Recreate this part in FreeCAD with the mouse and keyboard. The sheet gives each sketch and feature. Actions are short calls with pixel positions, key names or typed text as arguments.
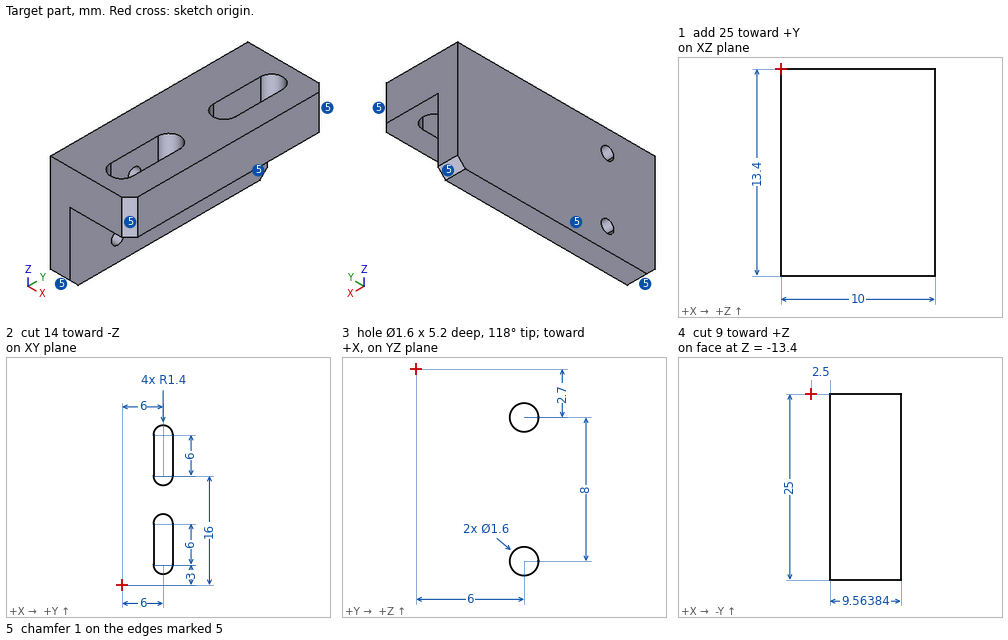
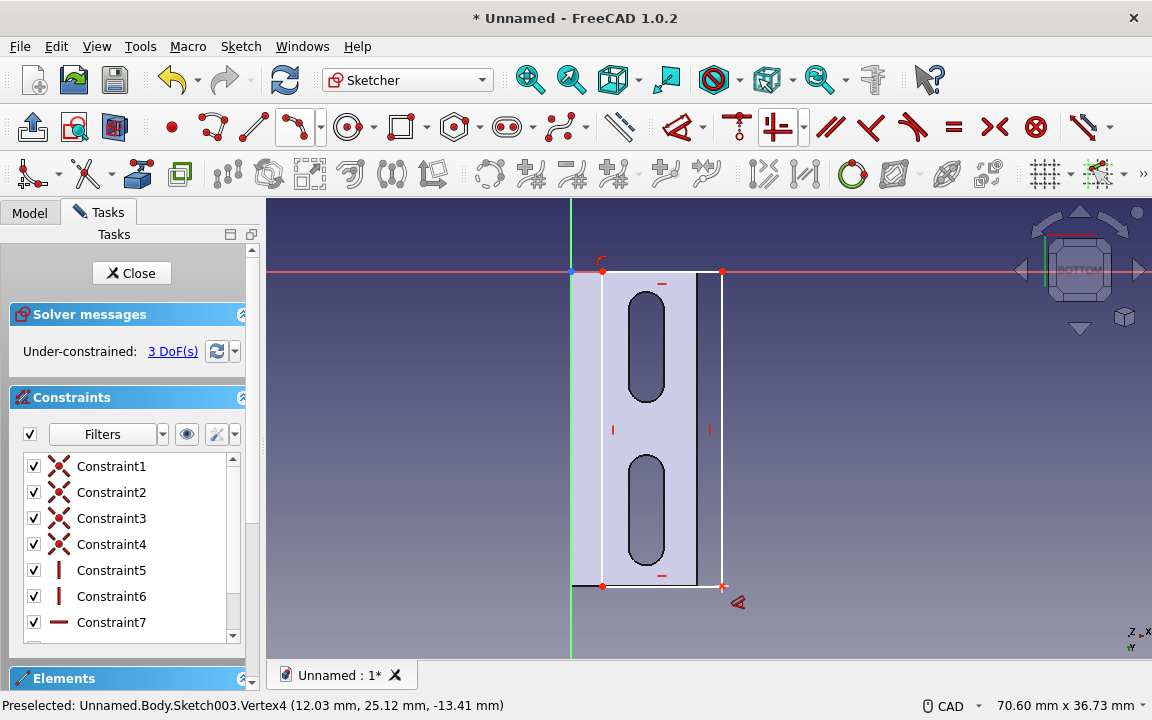
click(602, 366)
click(636, 429)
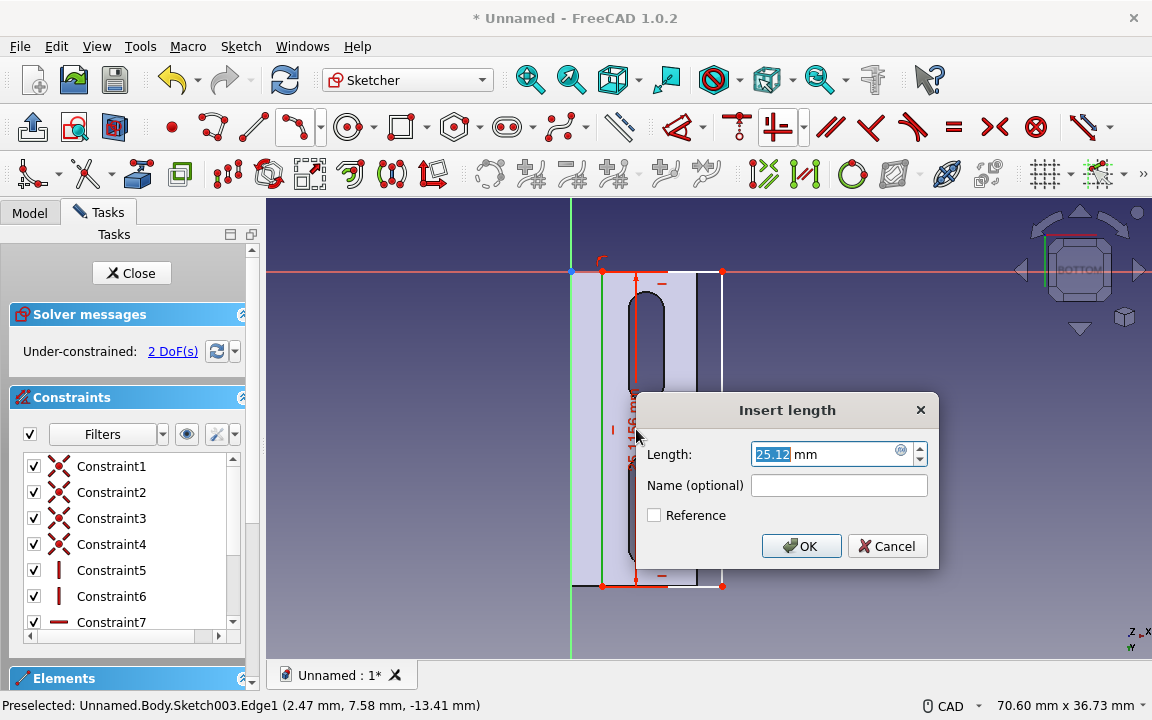
text(25)
key(Return)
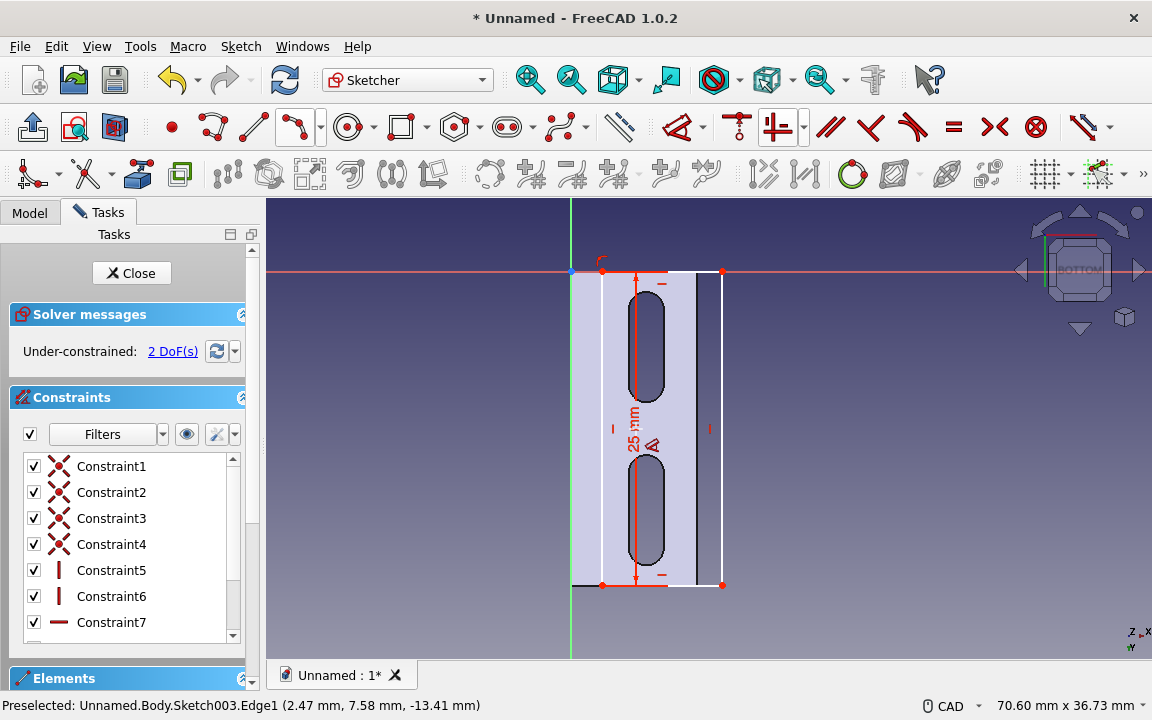
scroll(602, 272, up, 2)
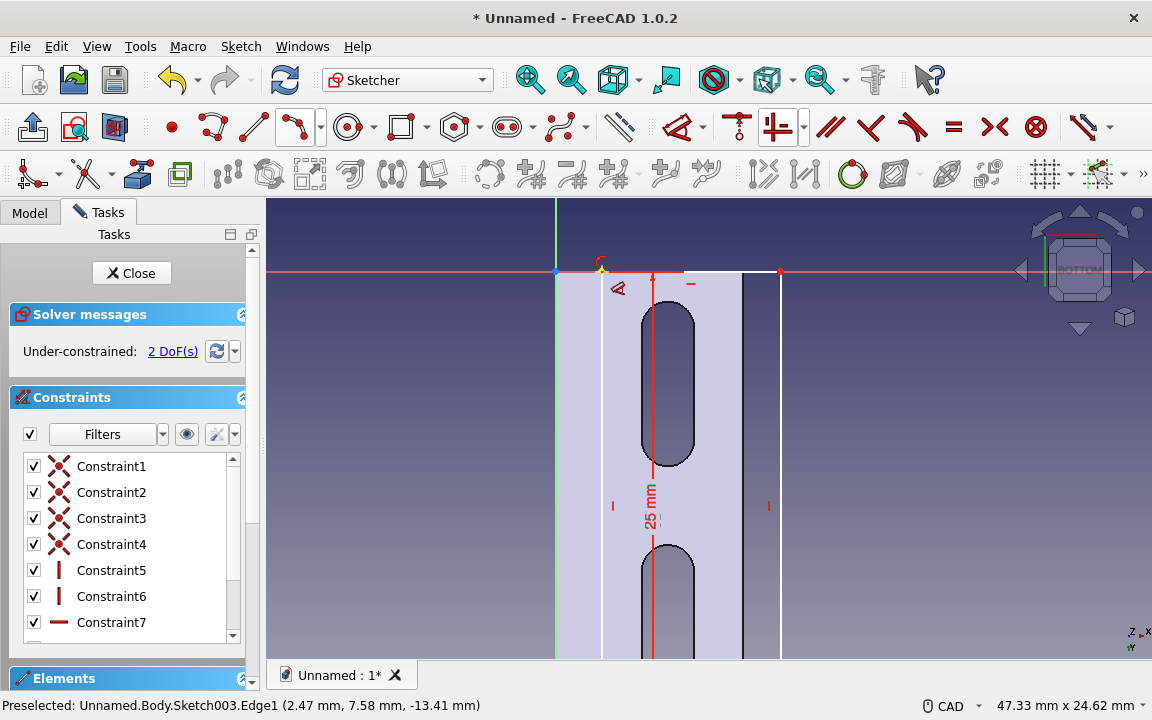
click(602, 272)
click(579, 238)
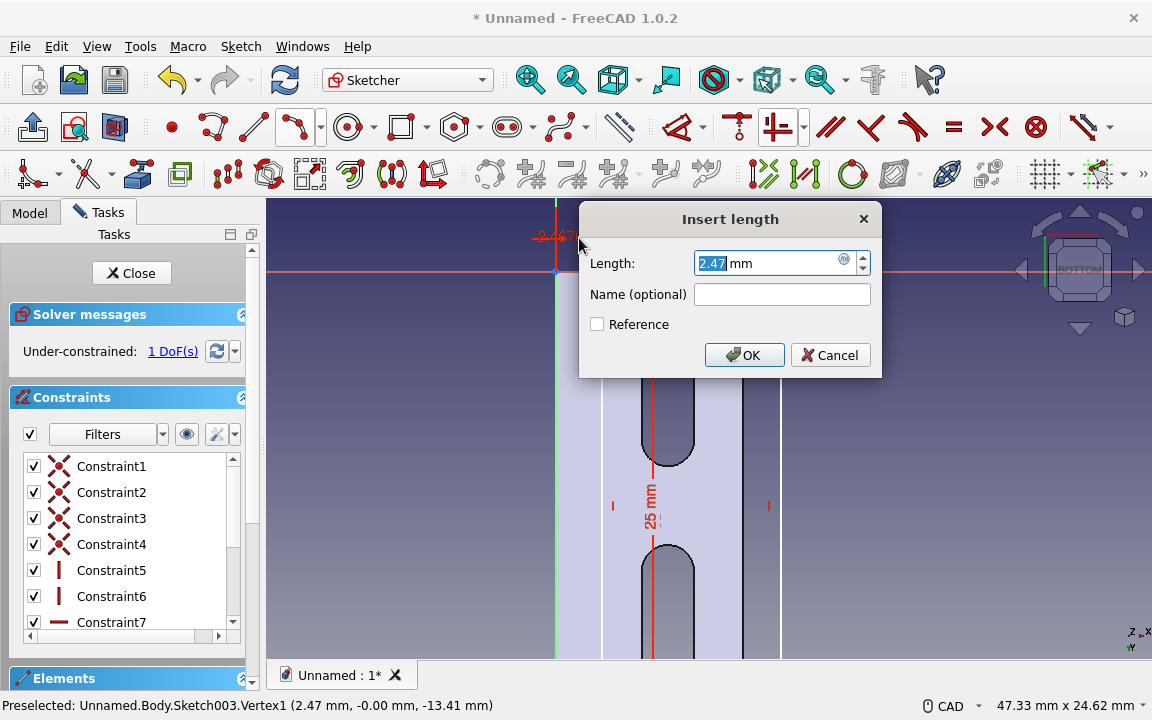
text(2.5)
key(Return)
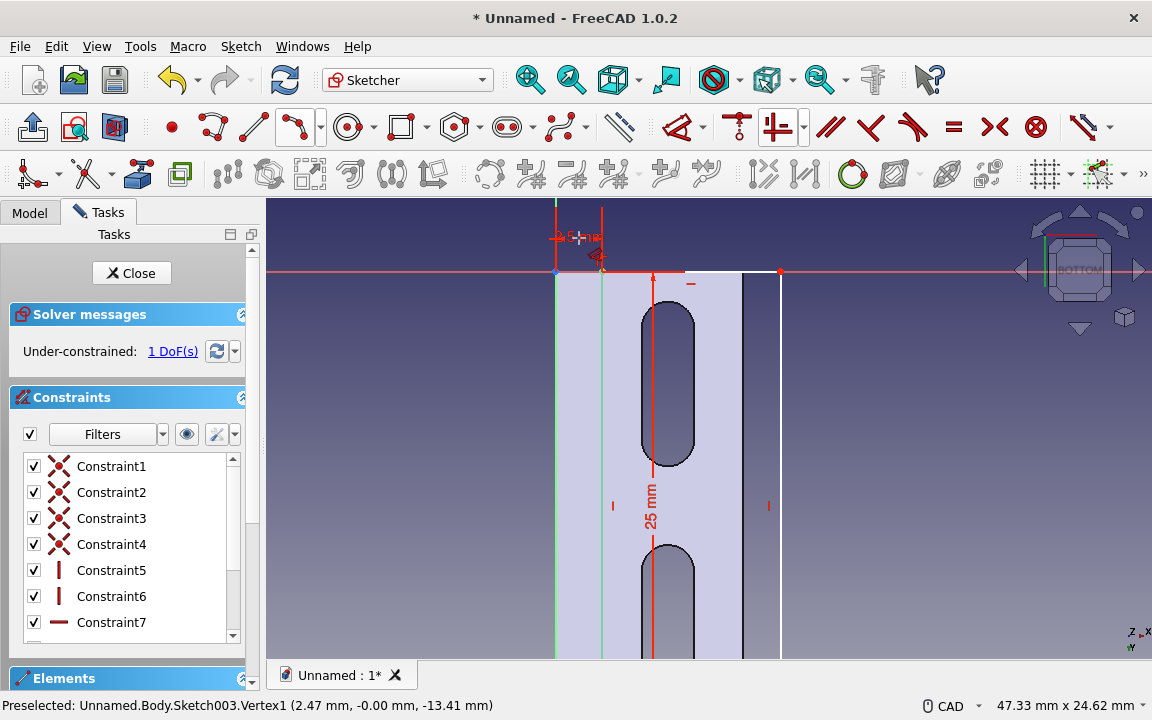
scroll(583, 272, down, 2)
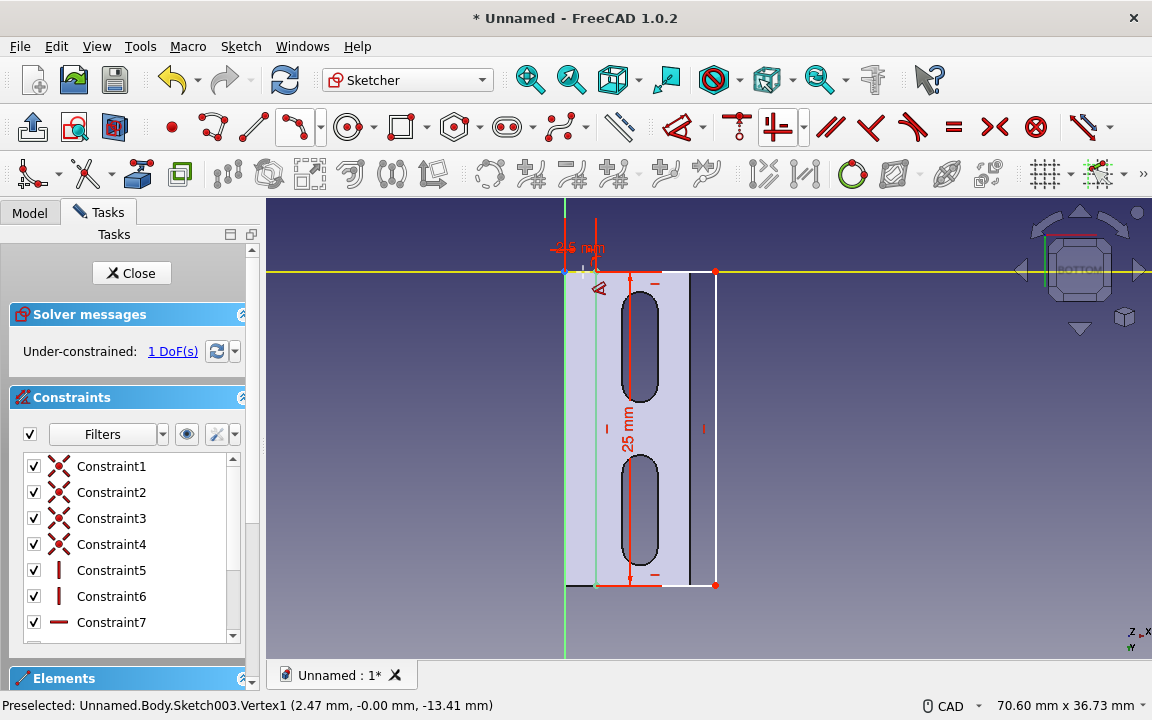
click(632, 586)
click(656, 620)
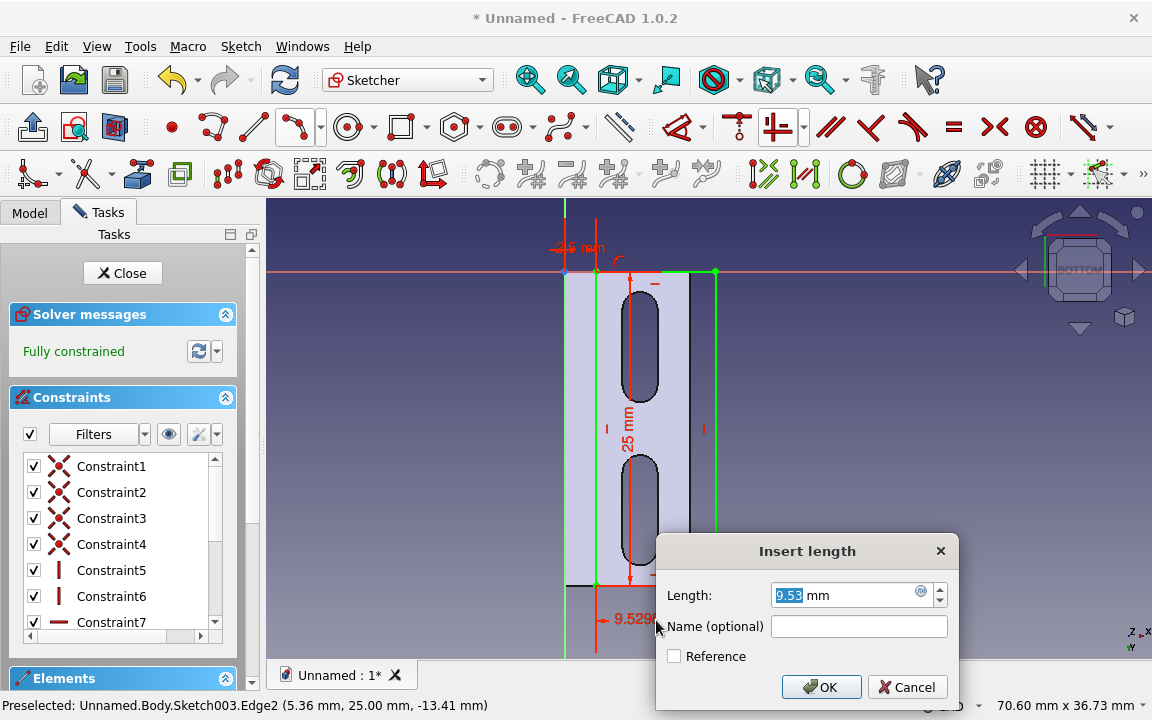
text(9.56384)
key(Return)
key(Escape)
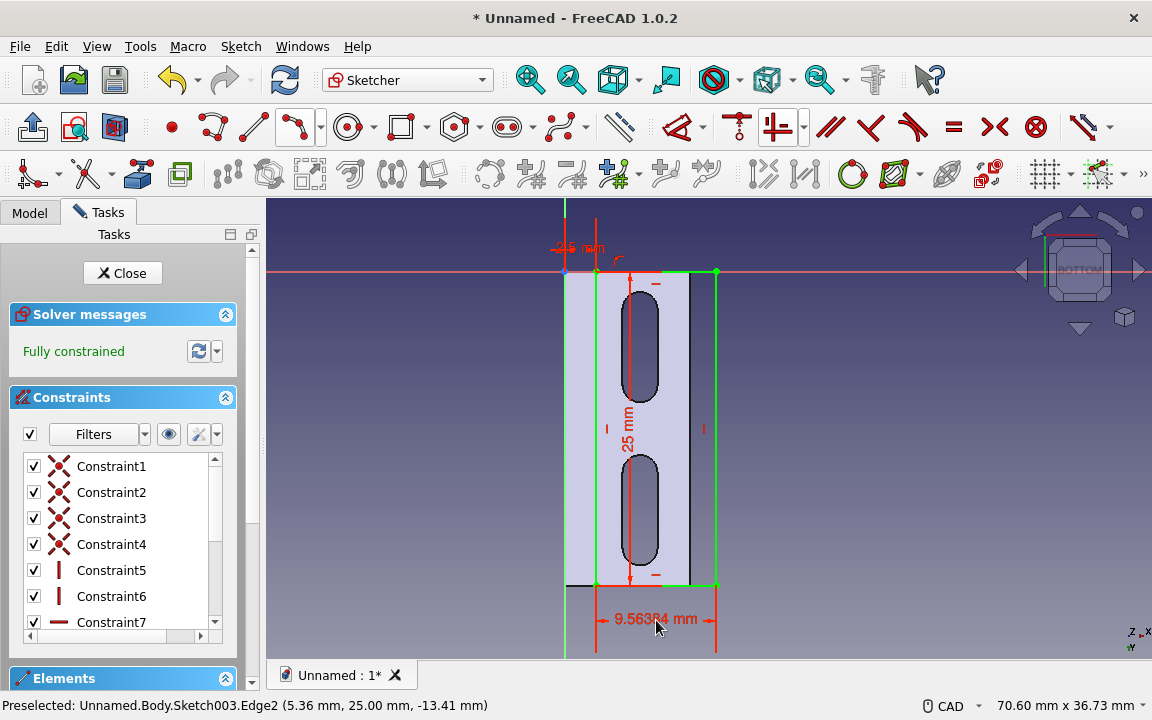
click(123, 273)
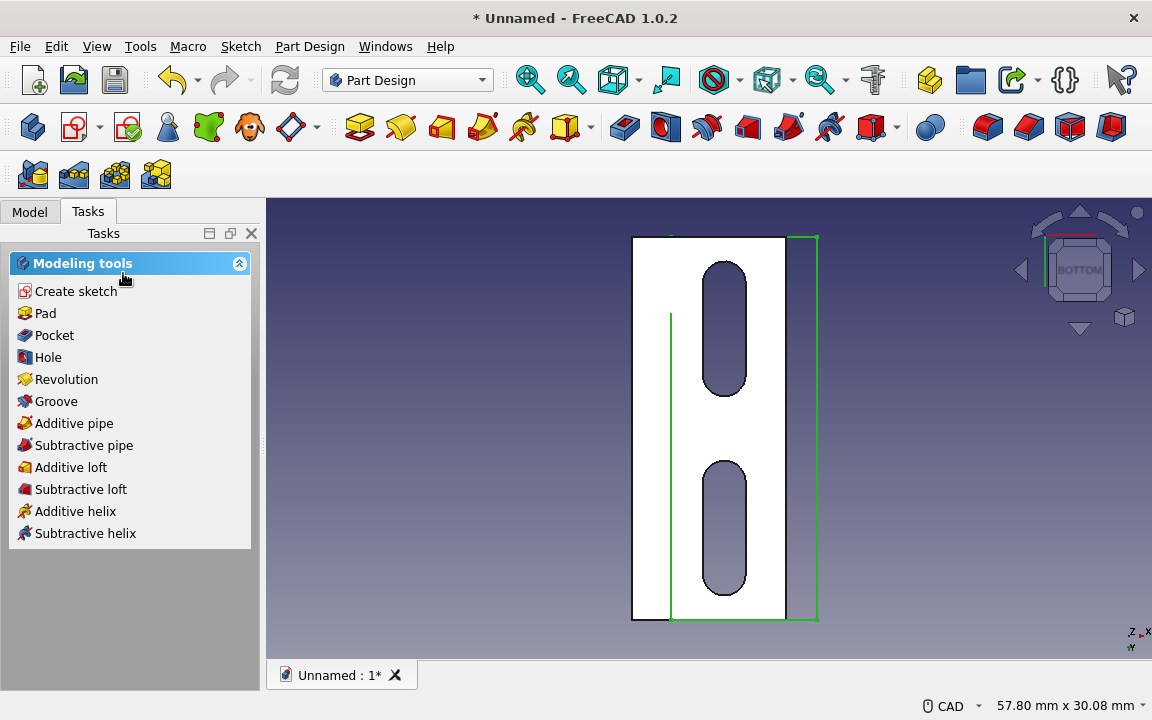
click(625, 128)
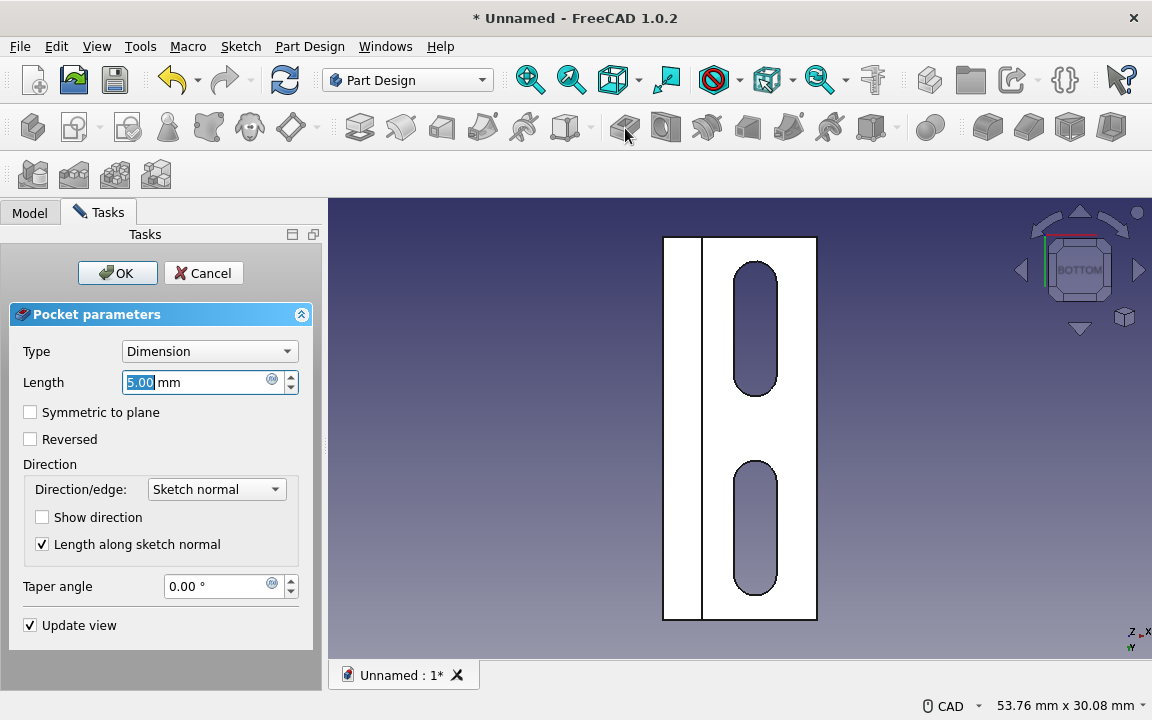
text(9)
key(Tab)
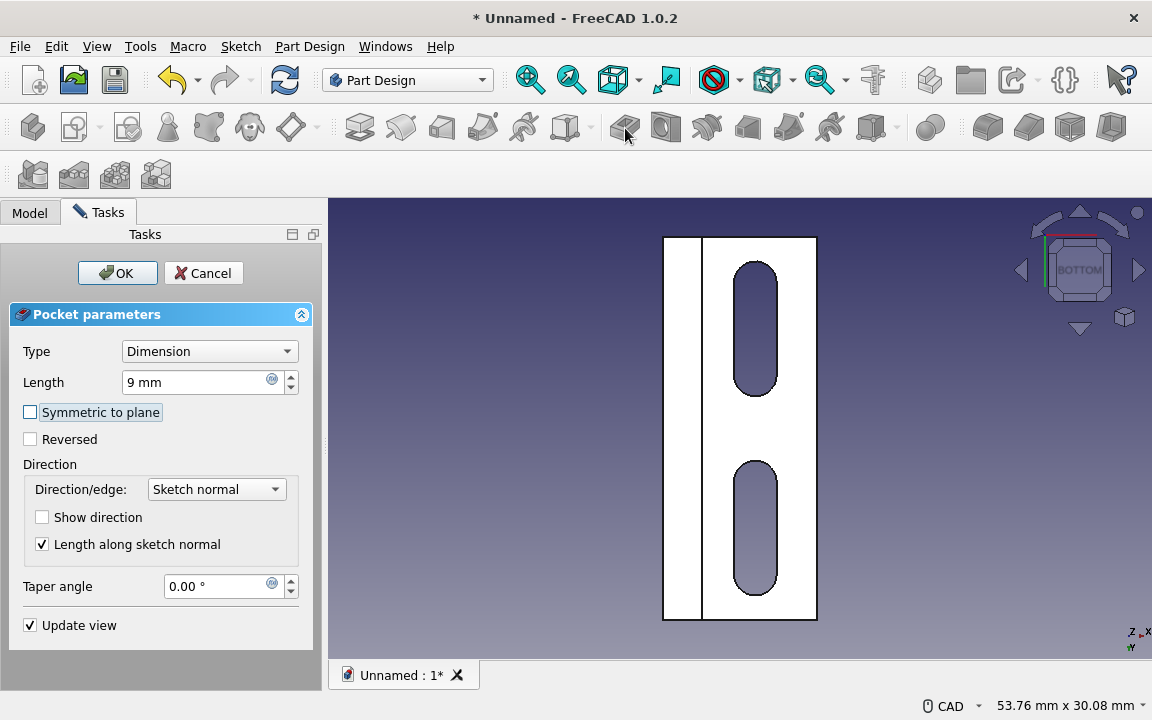
click(118, 273)